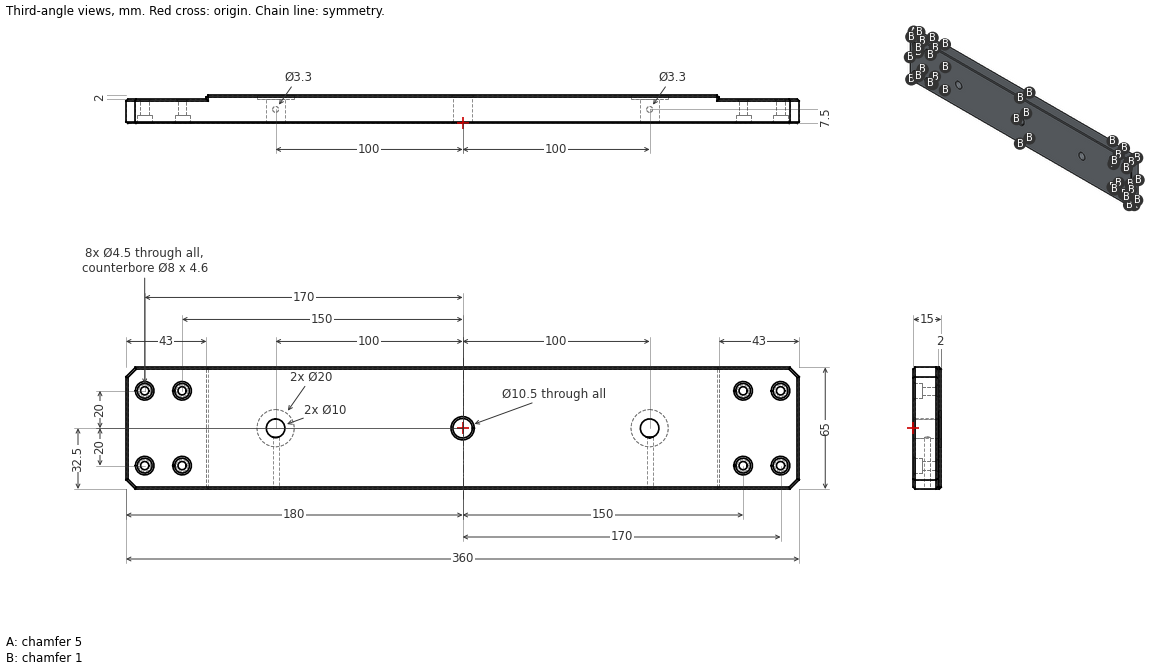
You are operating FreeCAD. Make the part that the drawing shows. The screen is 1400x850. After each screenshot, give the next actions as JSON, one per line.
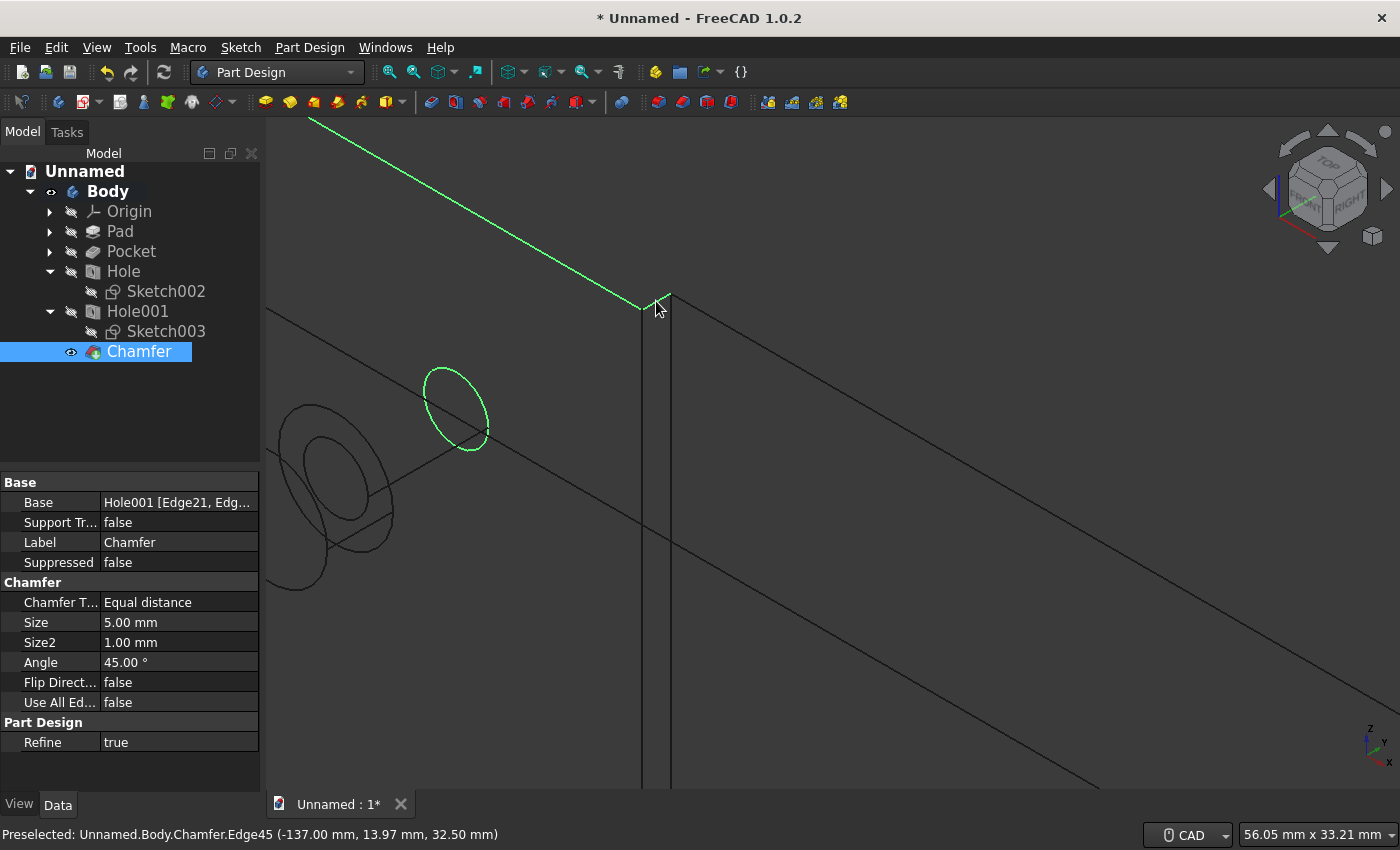
{"action": "key", "text": "v f"}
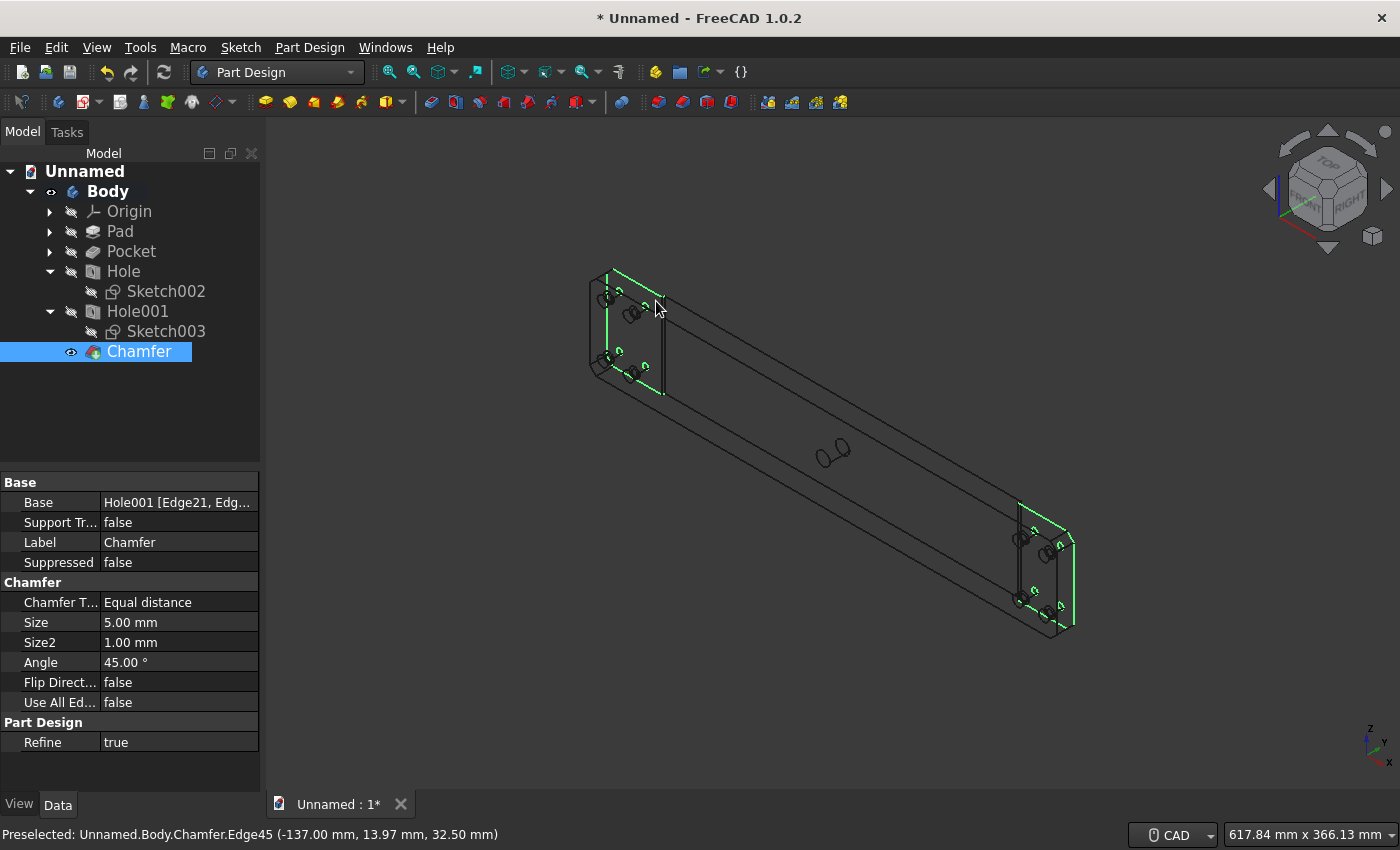
{"action": "key", "text": "2"}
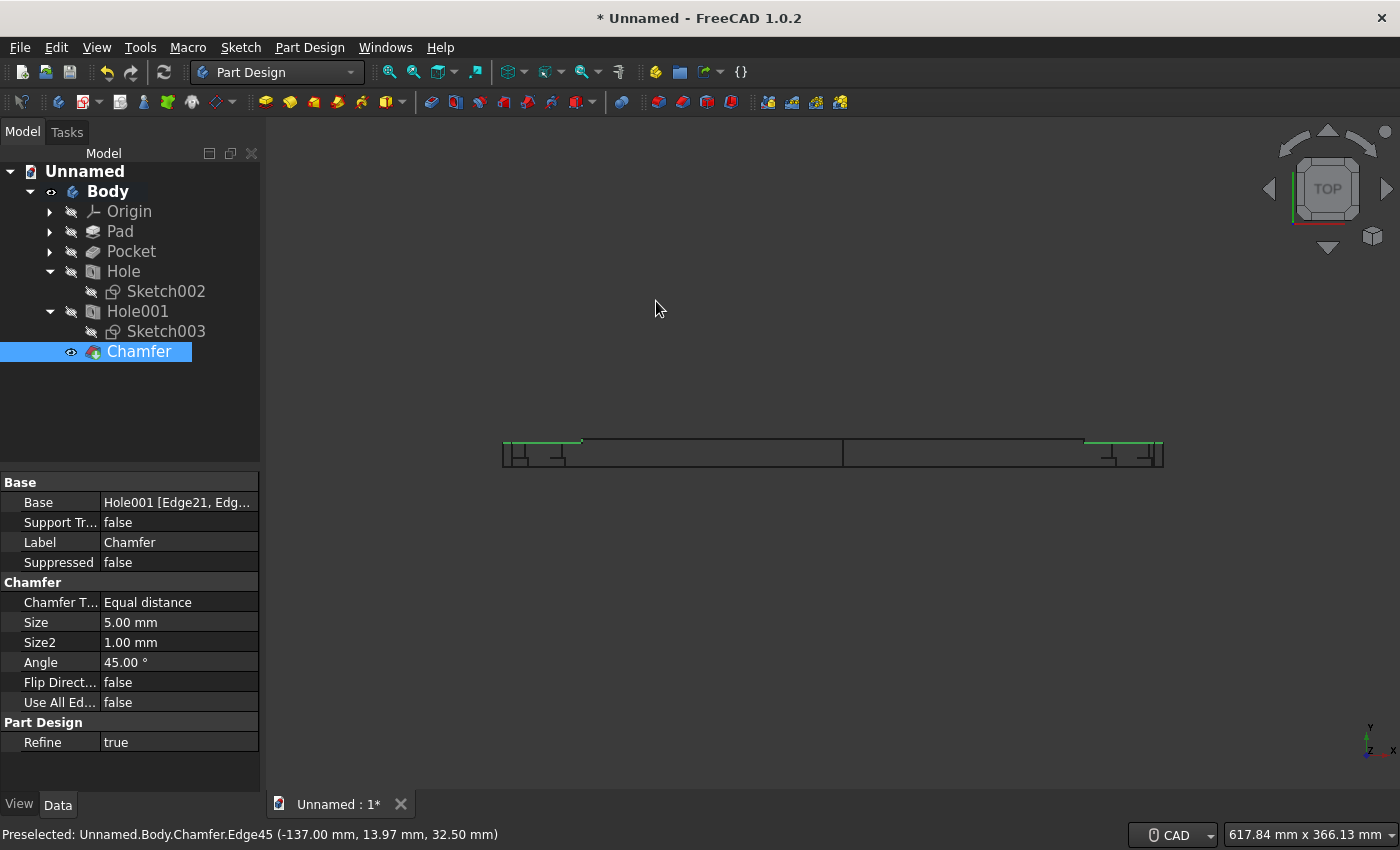
{"action": "scroll", "coordinate": [1084, 440], "scroll_direction": "up", "scroll_amount": 12}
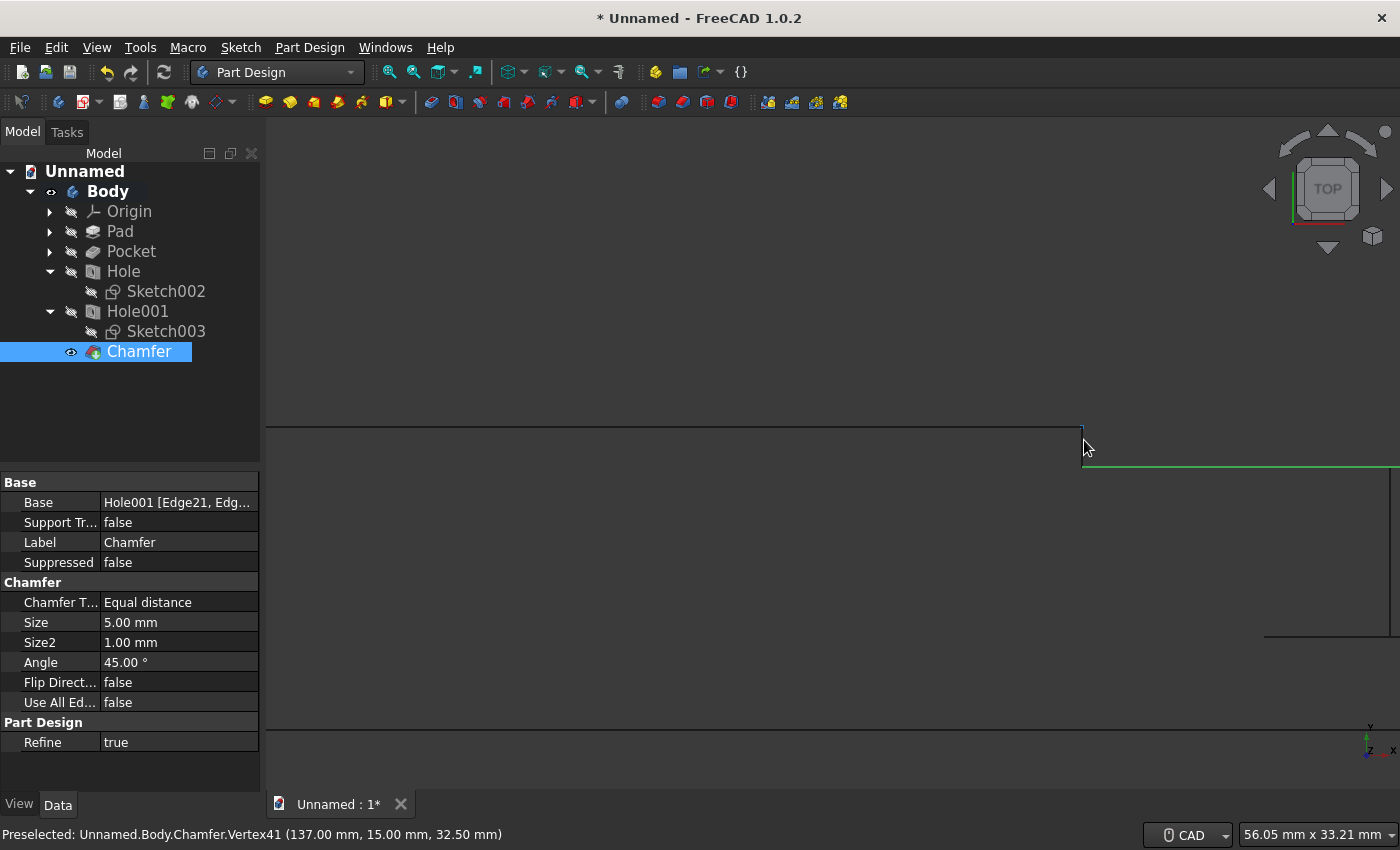
{"action": "left_click", "coordinate": [1082, 446], "text": "ctrl"}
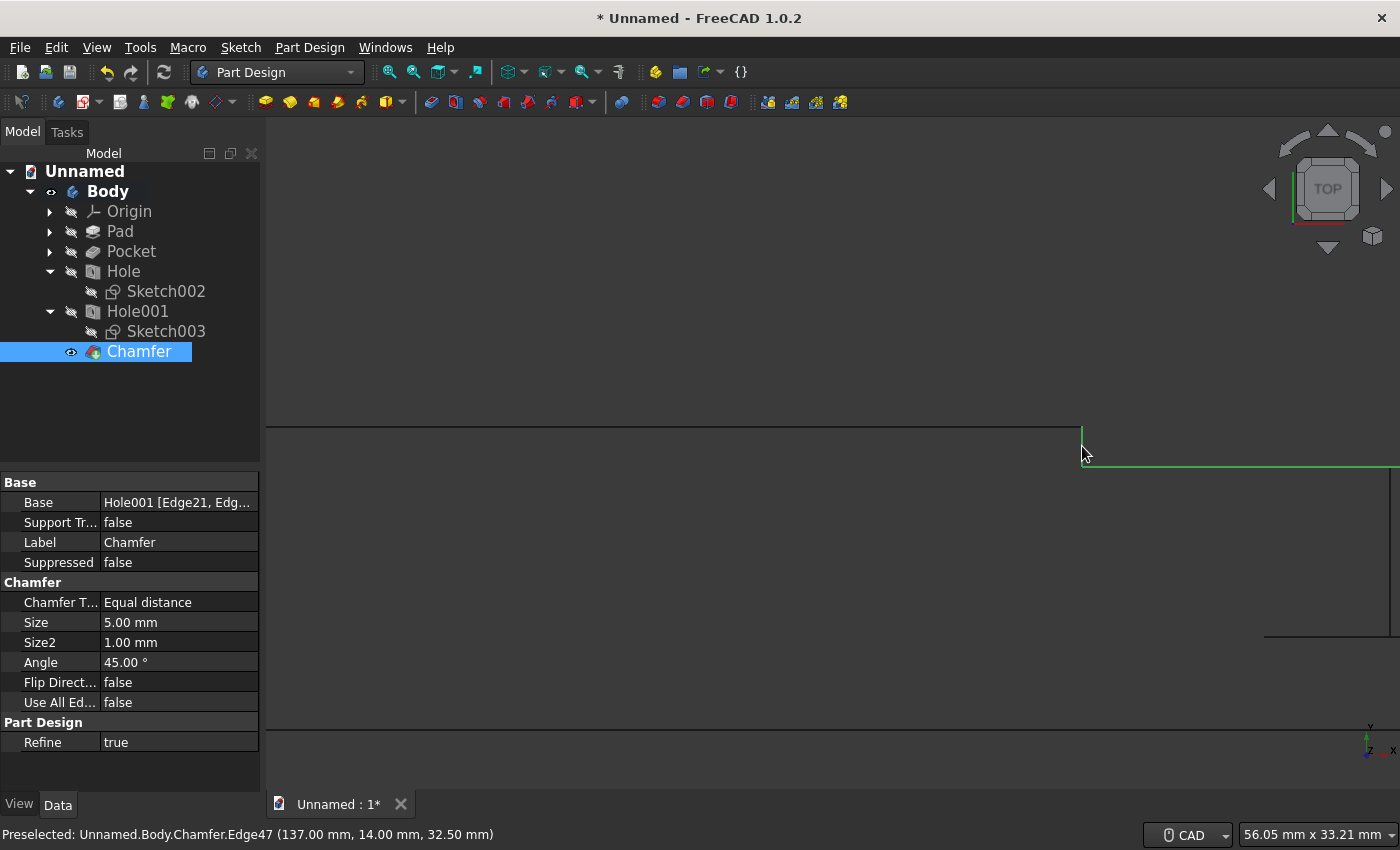
{"action": "key", "text": "v f"}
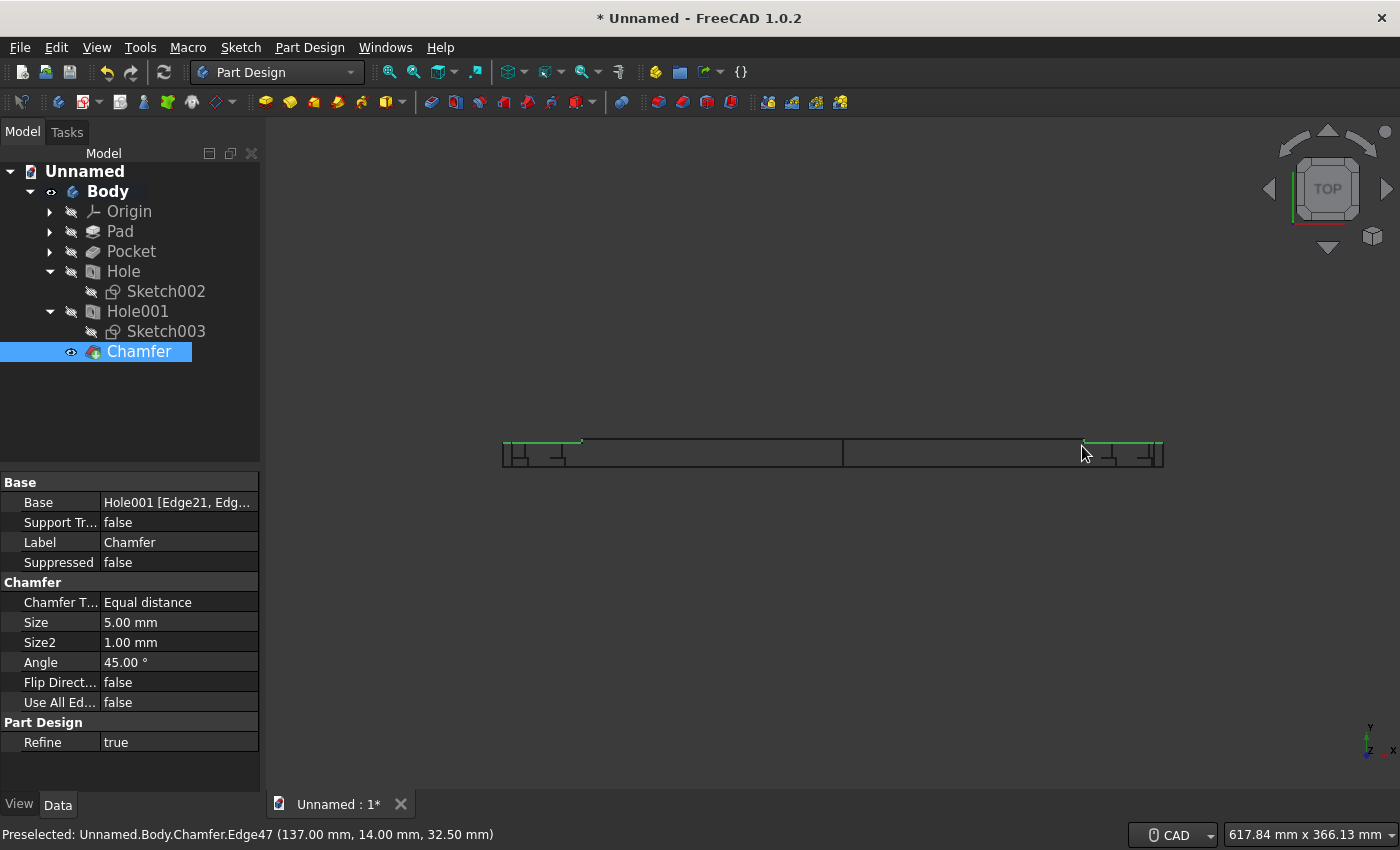
{"action": "key", "text": "1"}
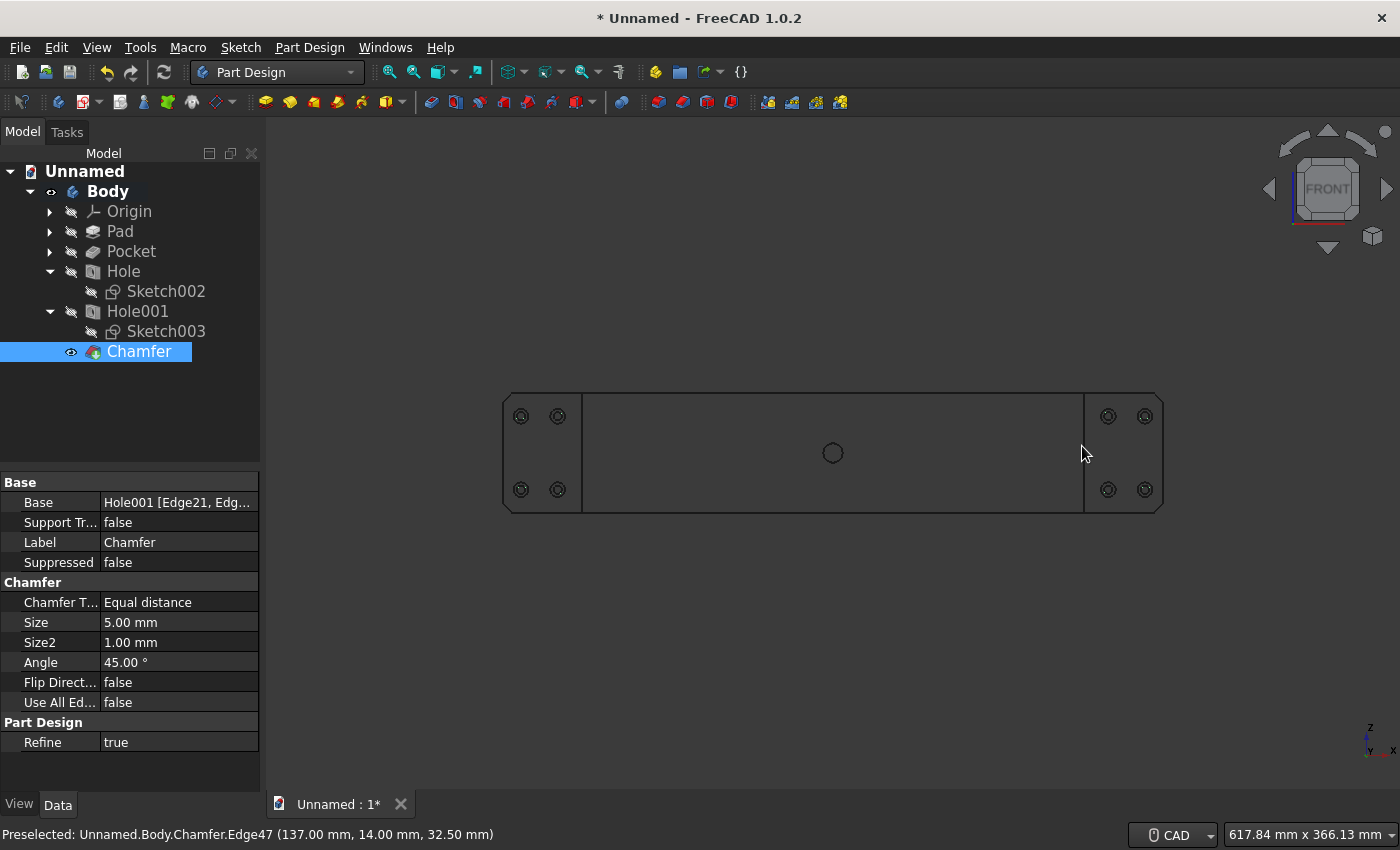
{"action": "scroll", "coordinate": [1084, 512], "scroll_direction": "up", "scroll_amount": 12}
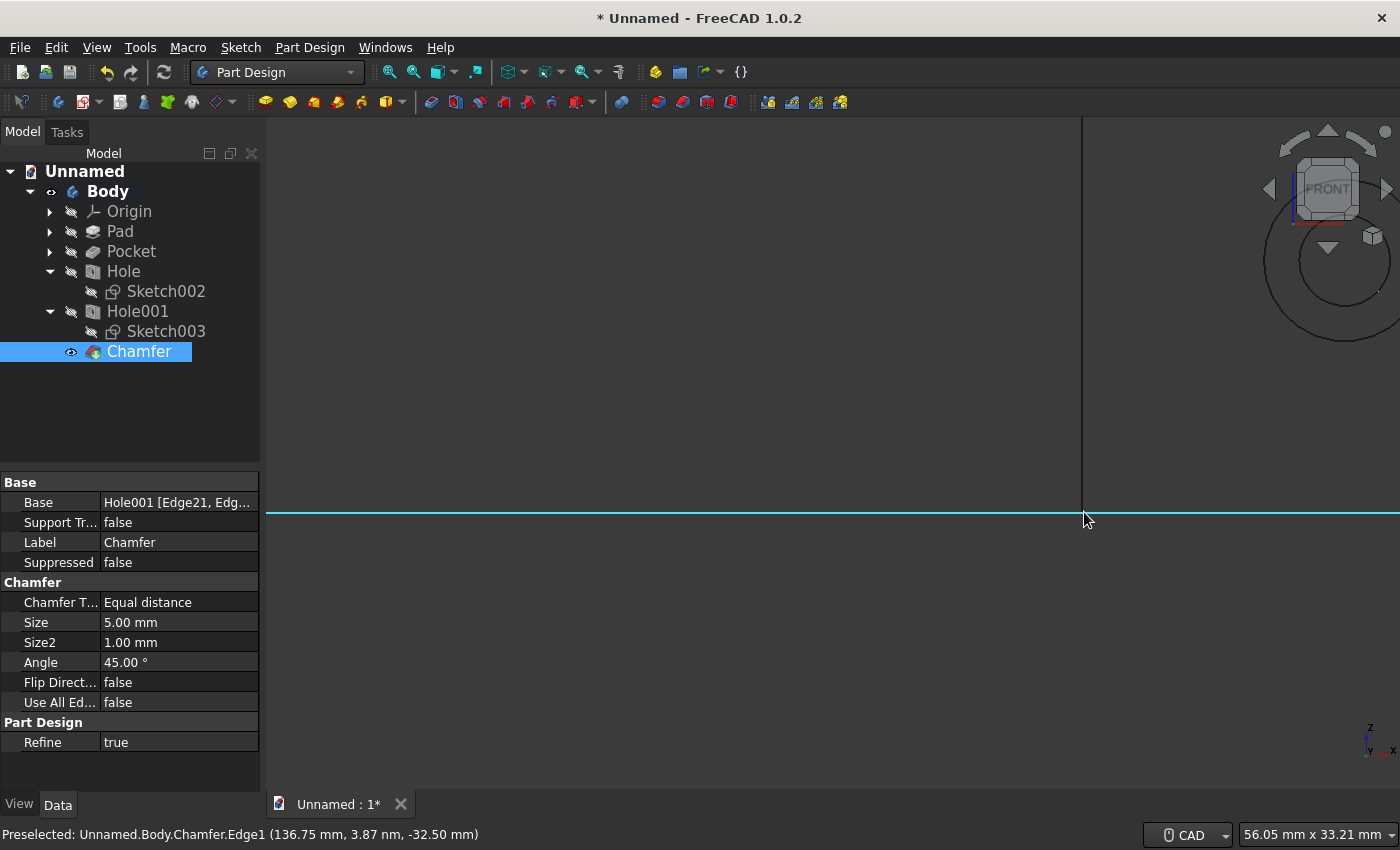
{"action": "left_click", "coordinate": [390, 72]}